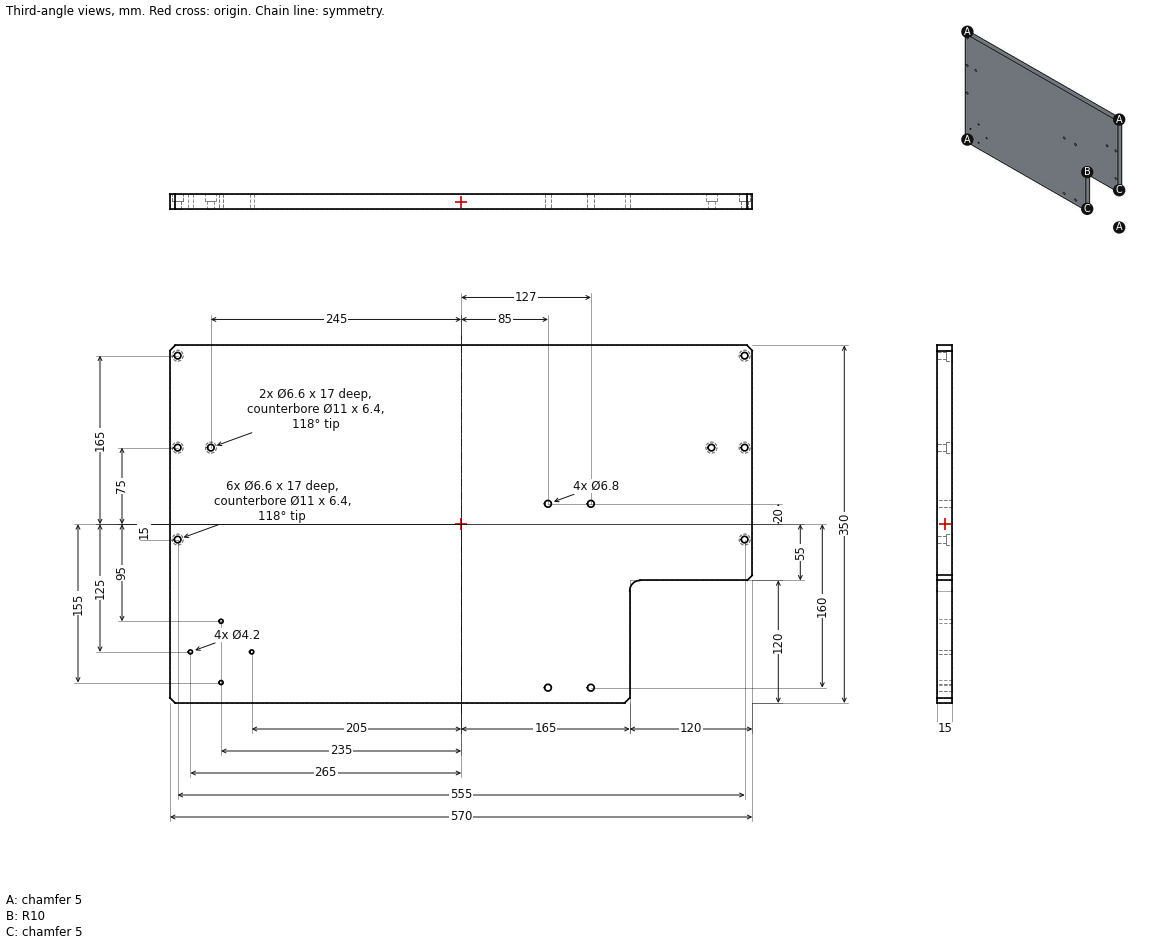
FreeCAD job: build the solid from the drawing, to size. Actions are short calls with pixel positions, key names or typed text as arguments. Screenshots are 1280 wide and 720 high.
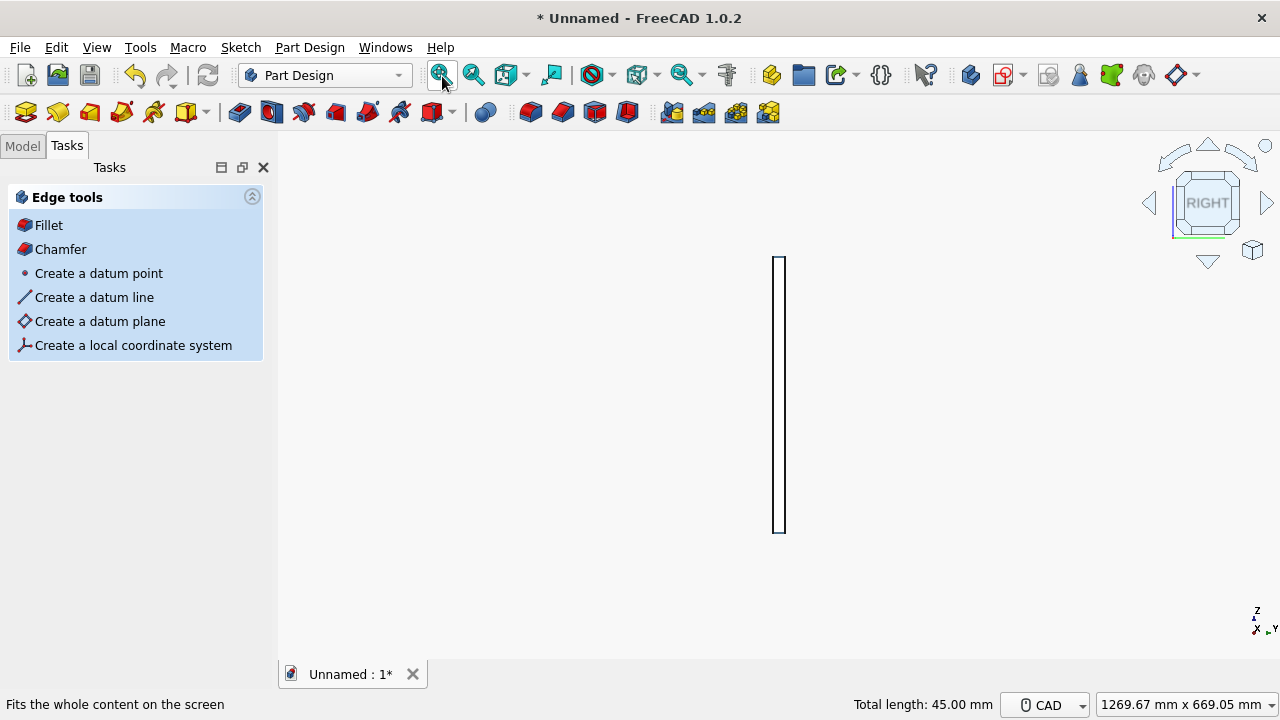
key(5)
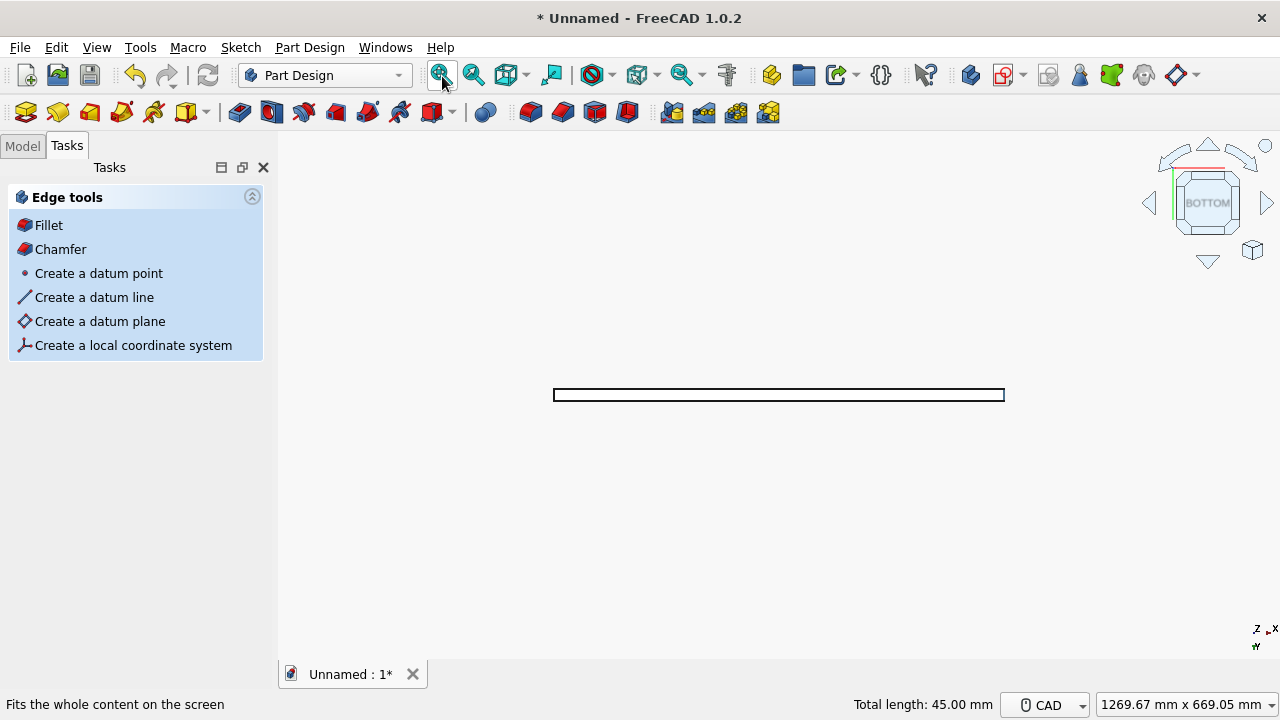
click(442, 76)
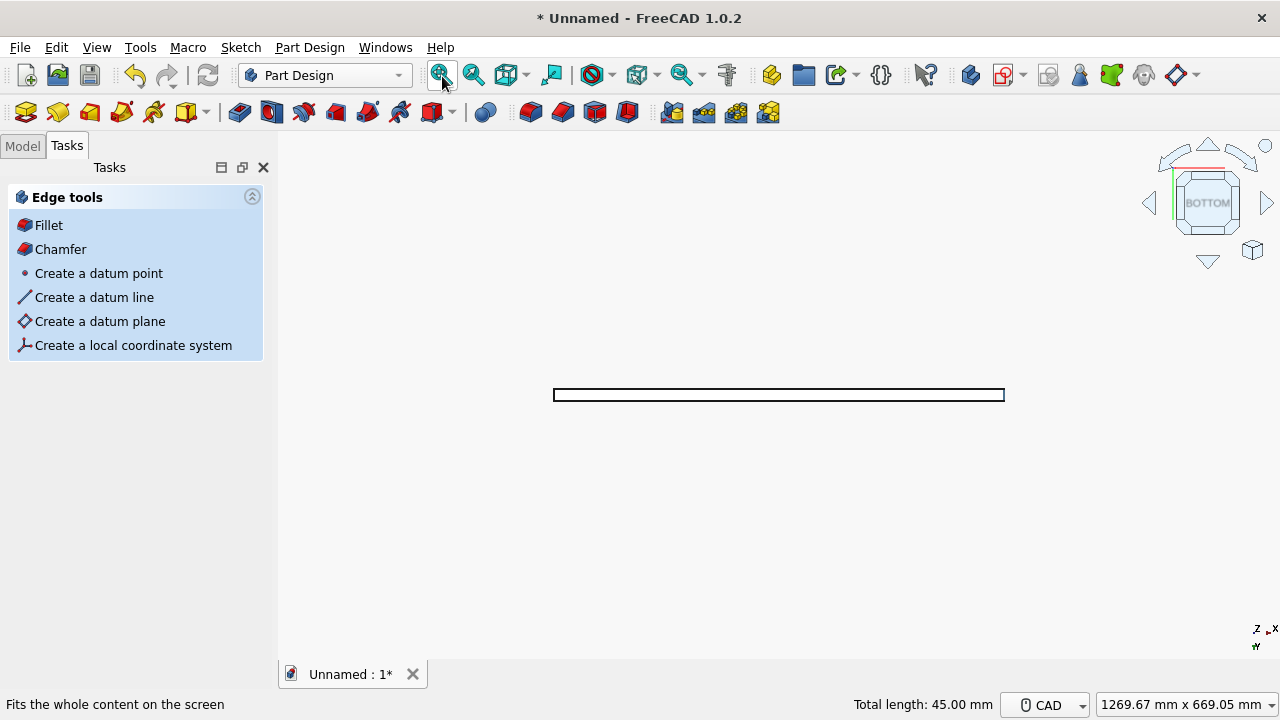
click(554, 395, ctrl)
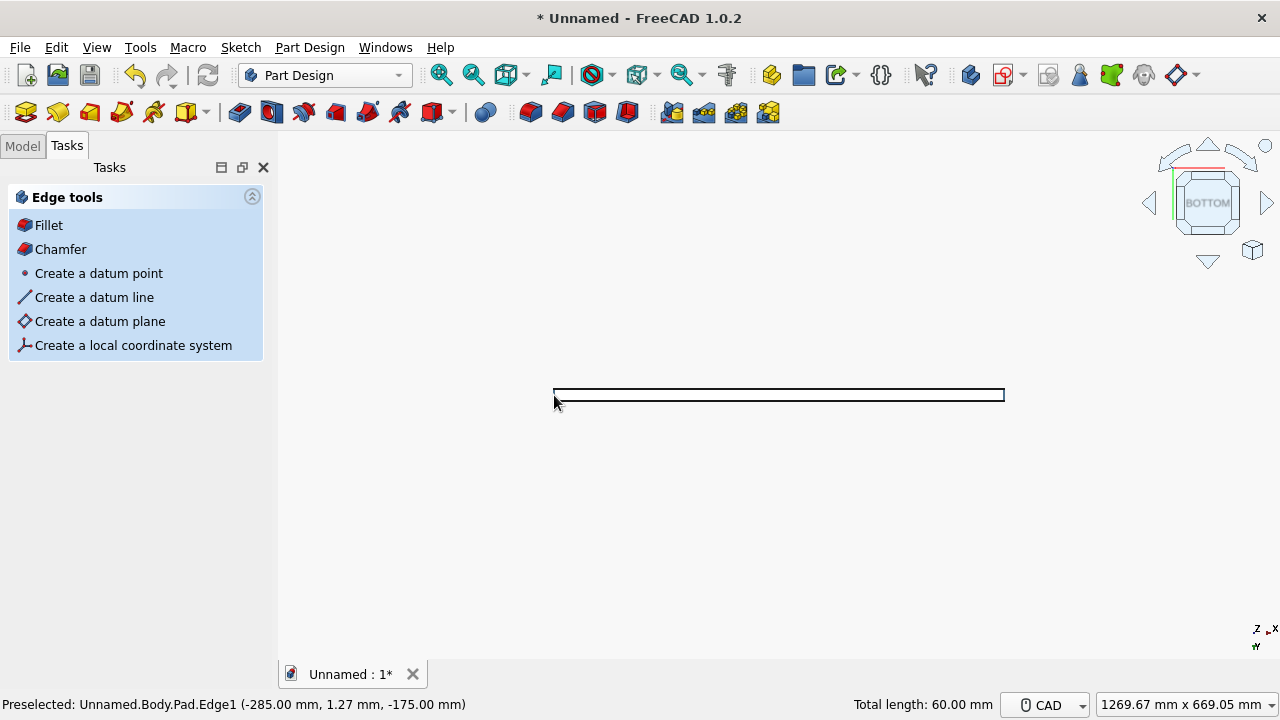
click(564, 112)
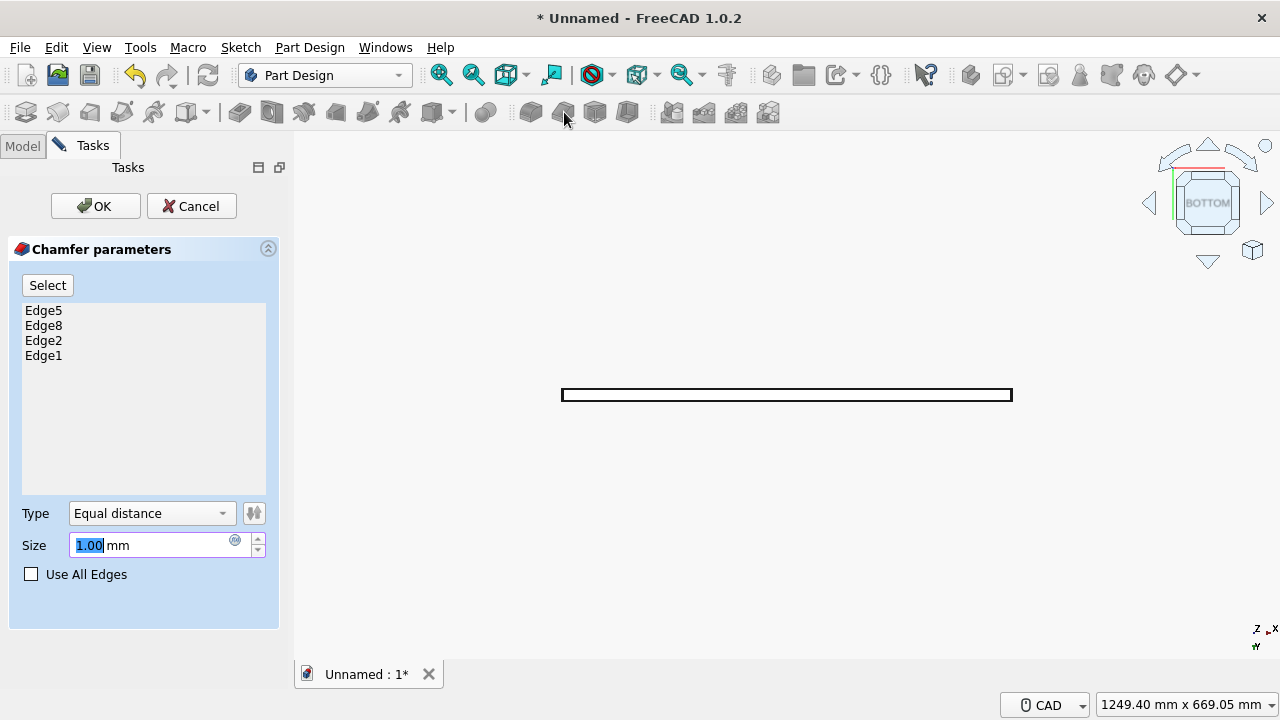
text(5)
key(Tab)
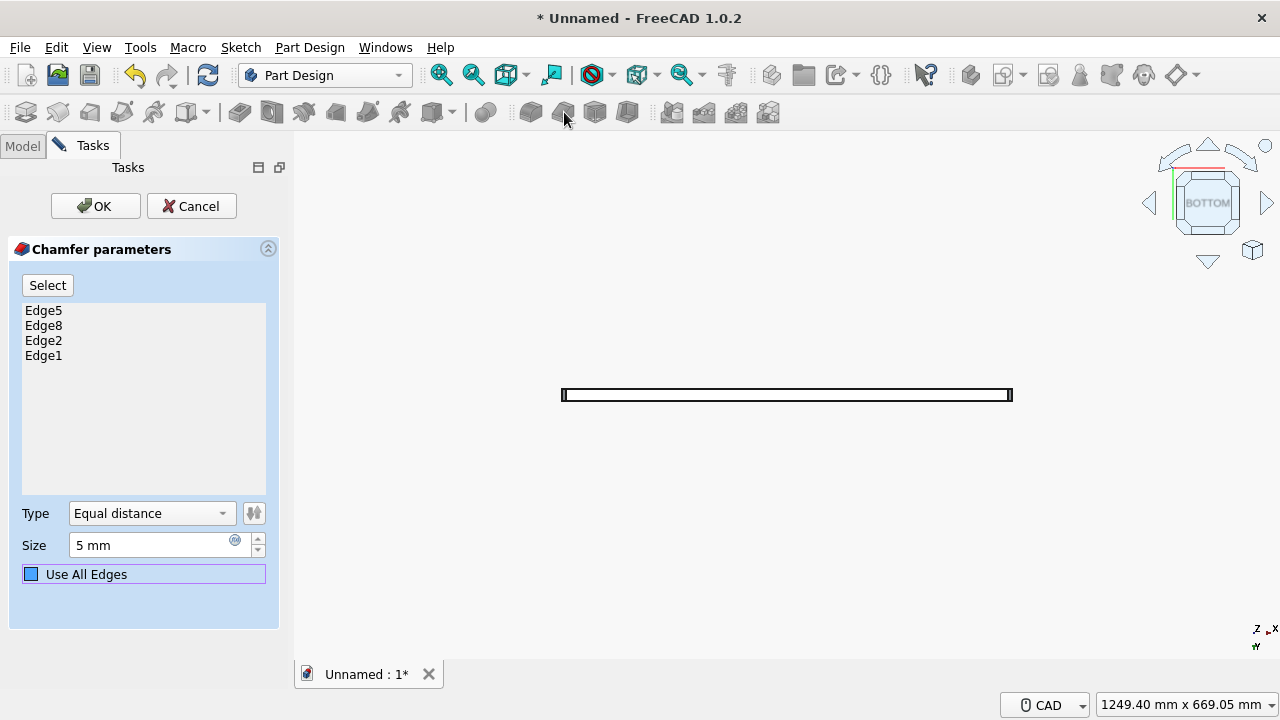
click(96, 206)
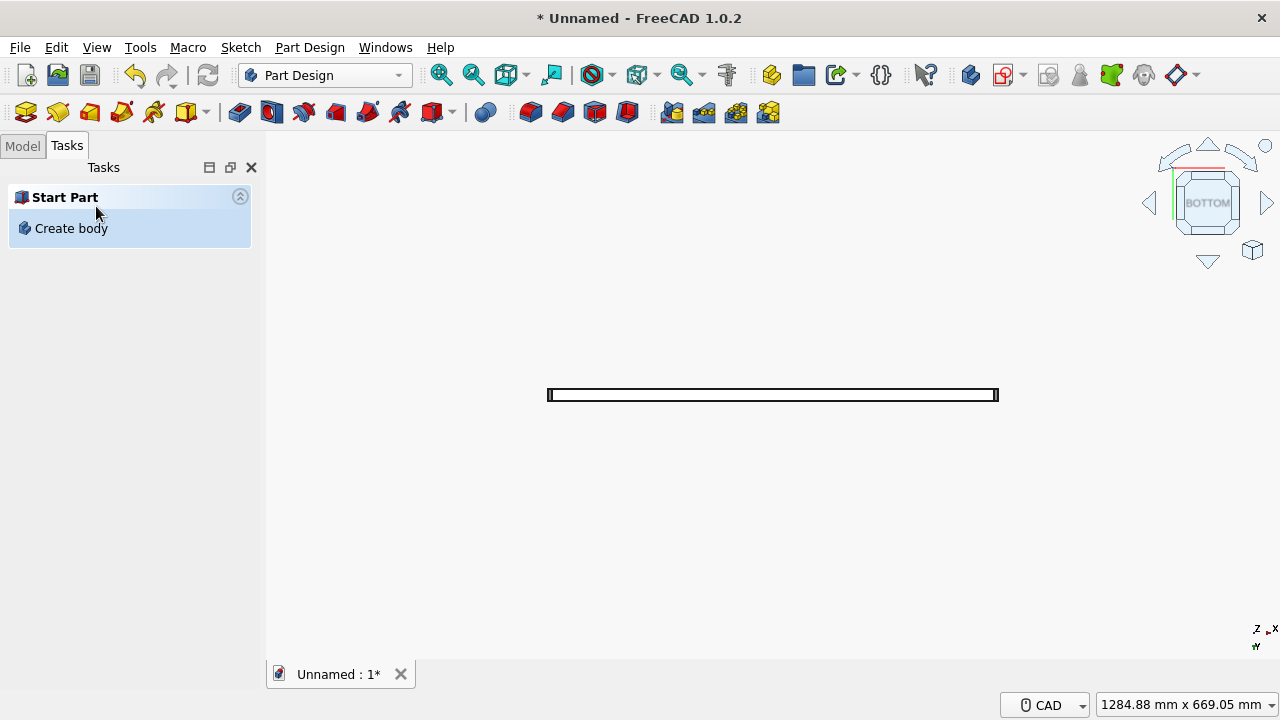
click(442, 76)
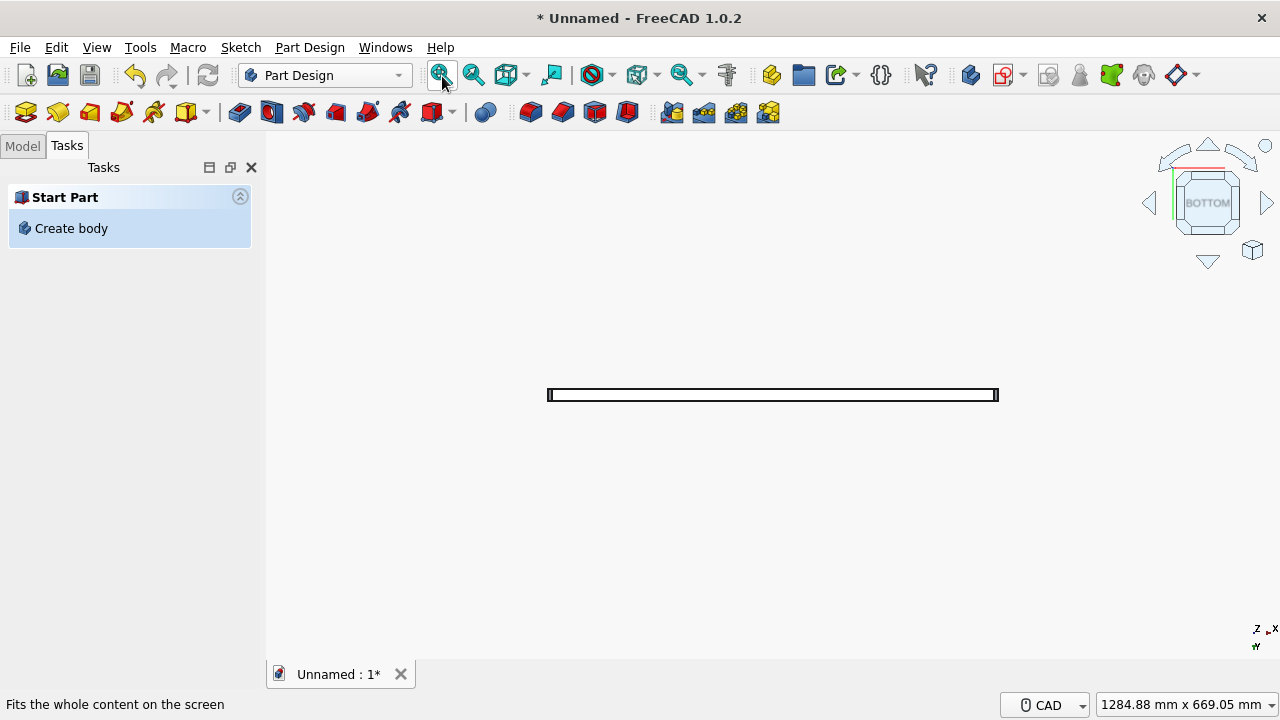
key(4)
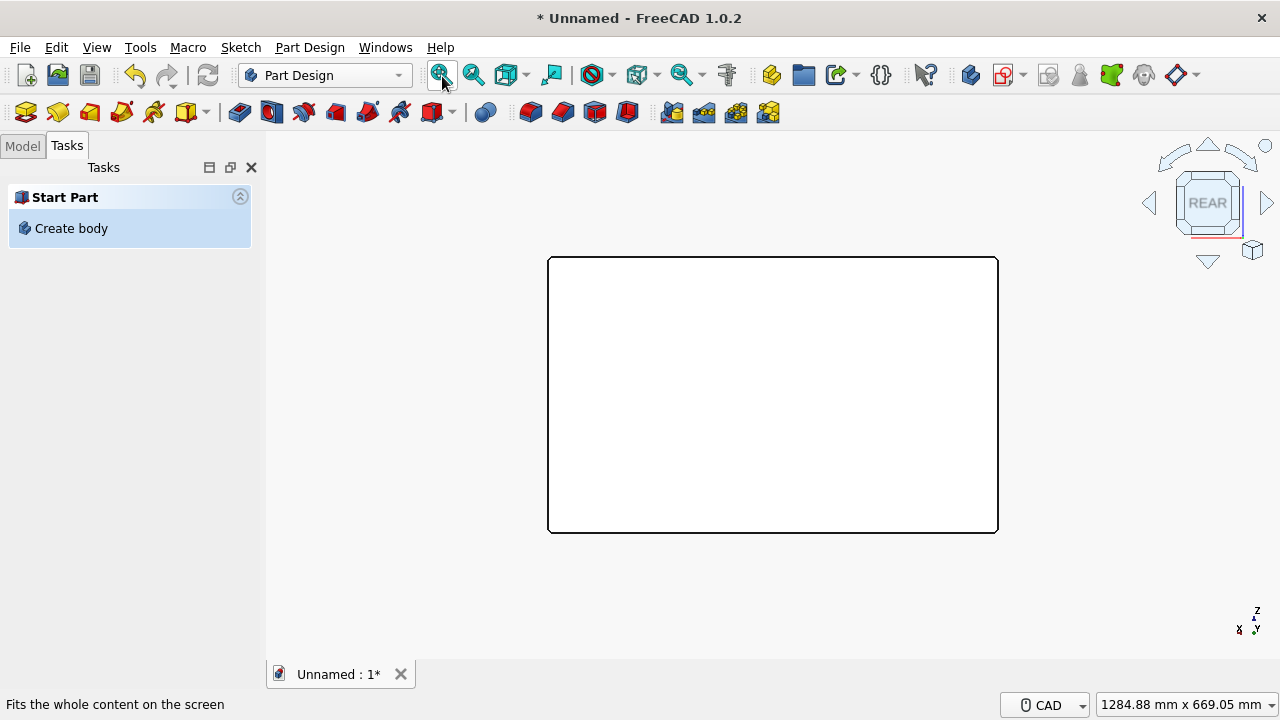
click(709, 394)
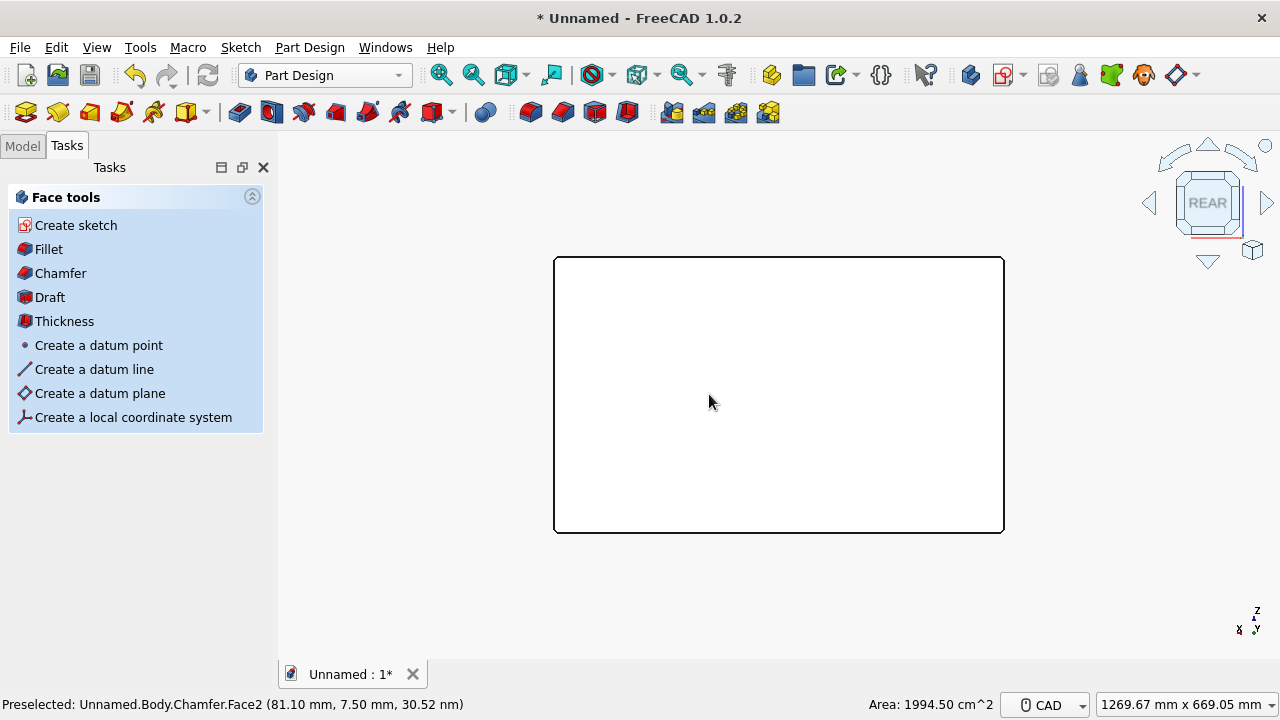
click(1004, 76)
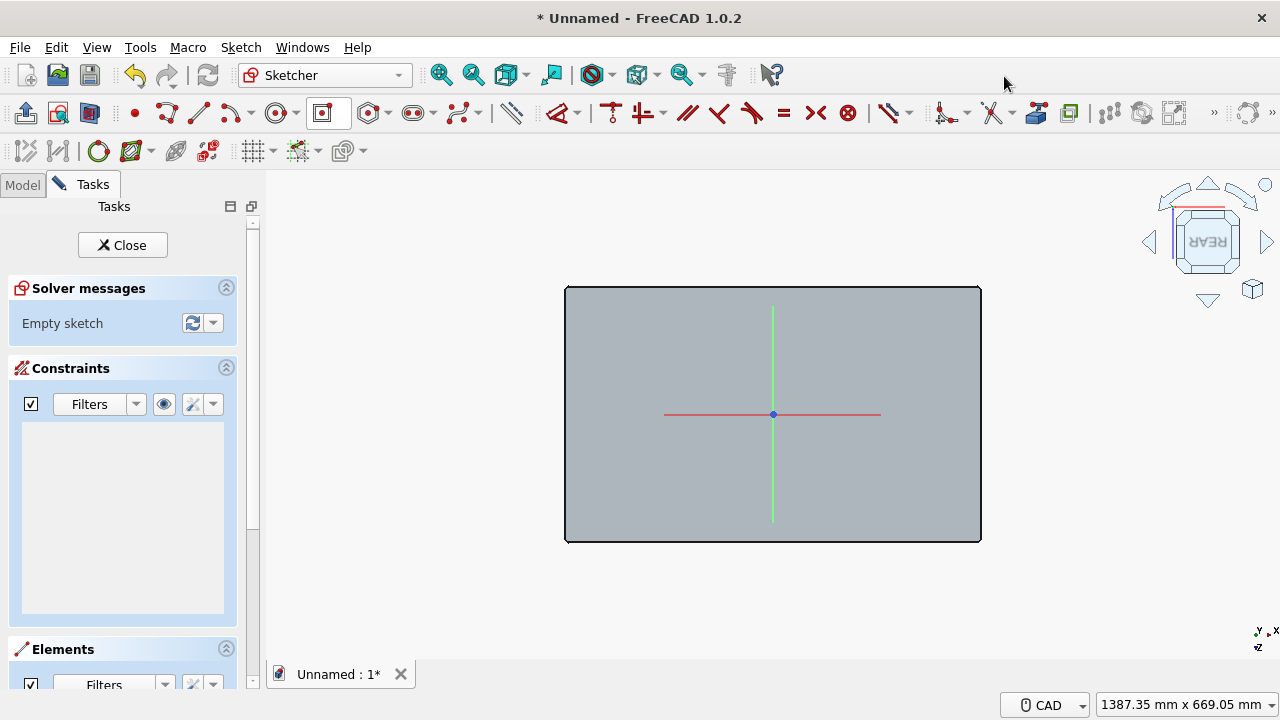
scroll(581, 305, up, 9)